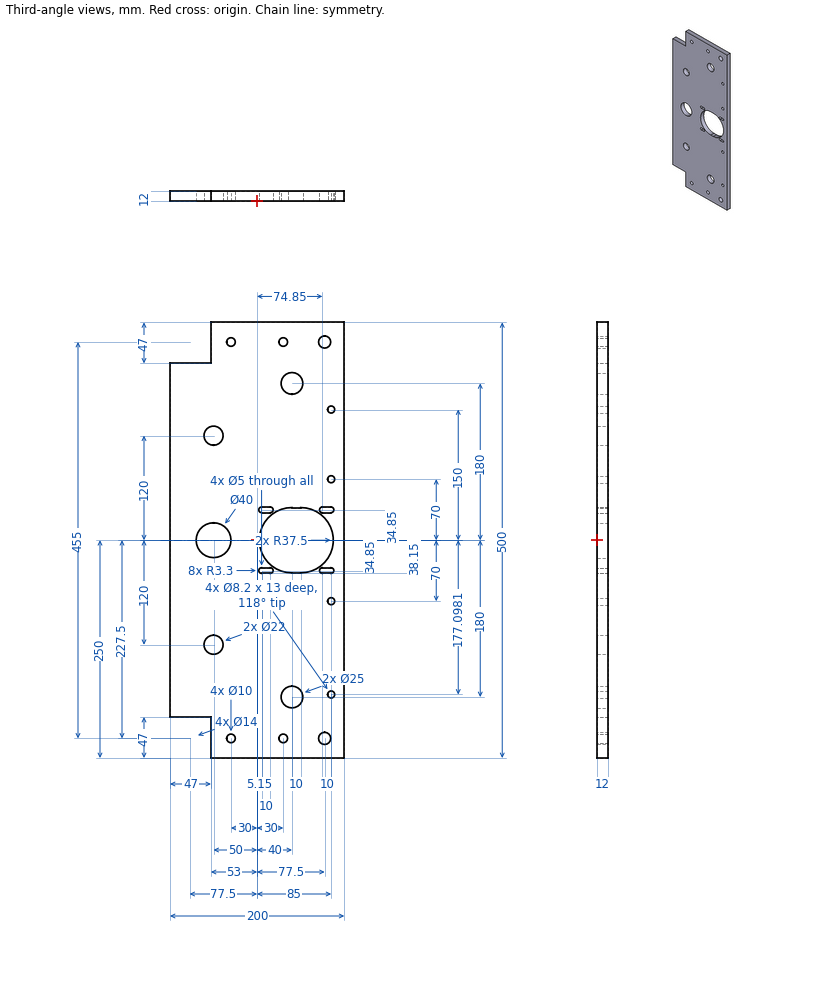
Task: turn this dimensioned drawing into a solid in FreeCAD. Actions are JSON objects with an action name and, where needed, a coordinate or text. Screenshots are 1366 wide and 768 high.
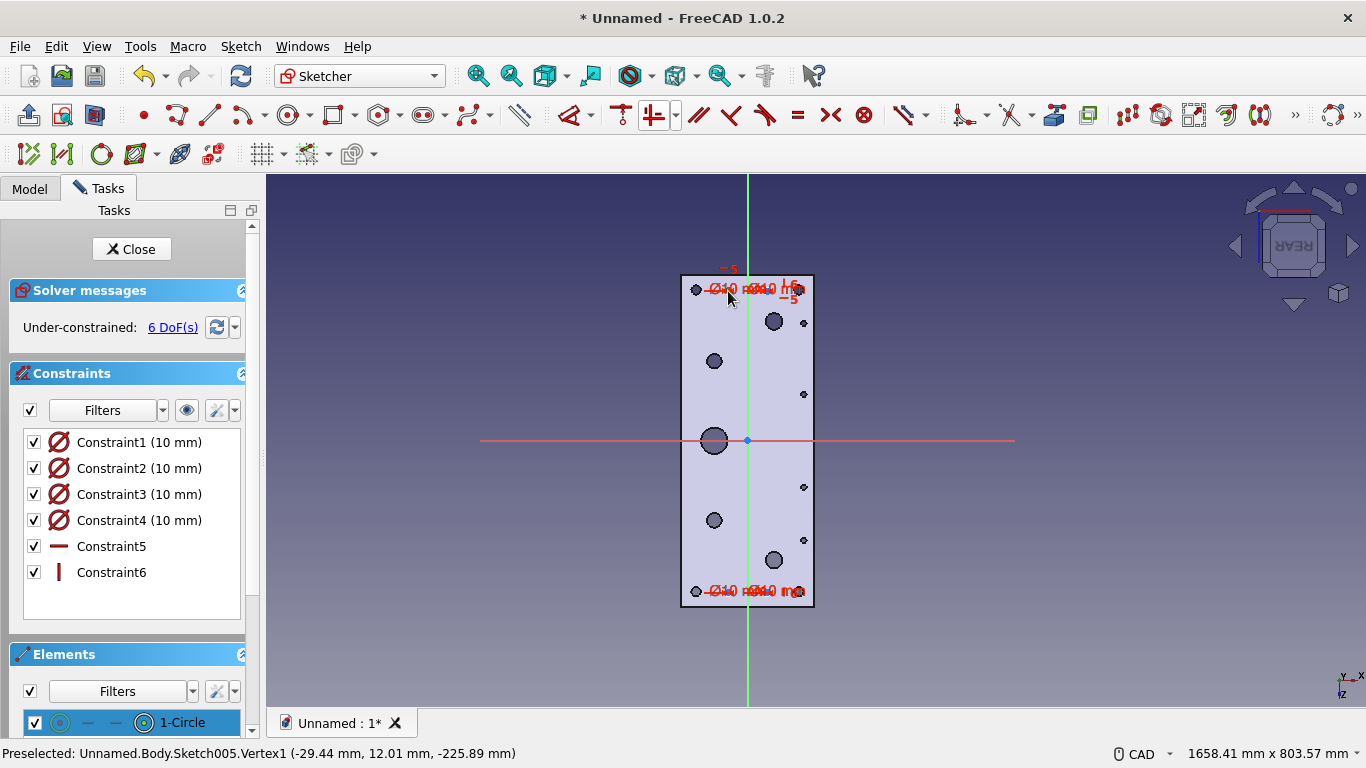
{"action": "left_click", "coordinate": [728, 593]}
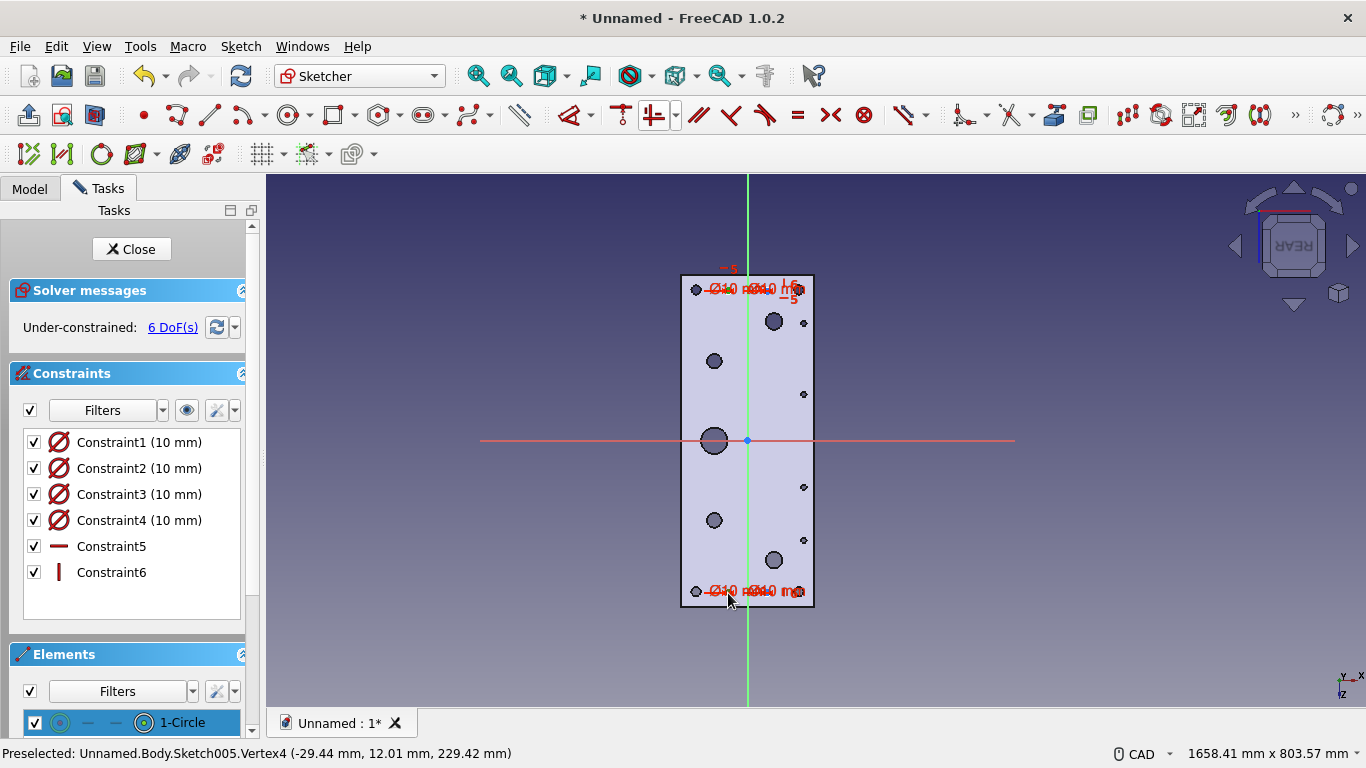
{"action": "key", "text": "v"}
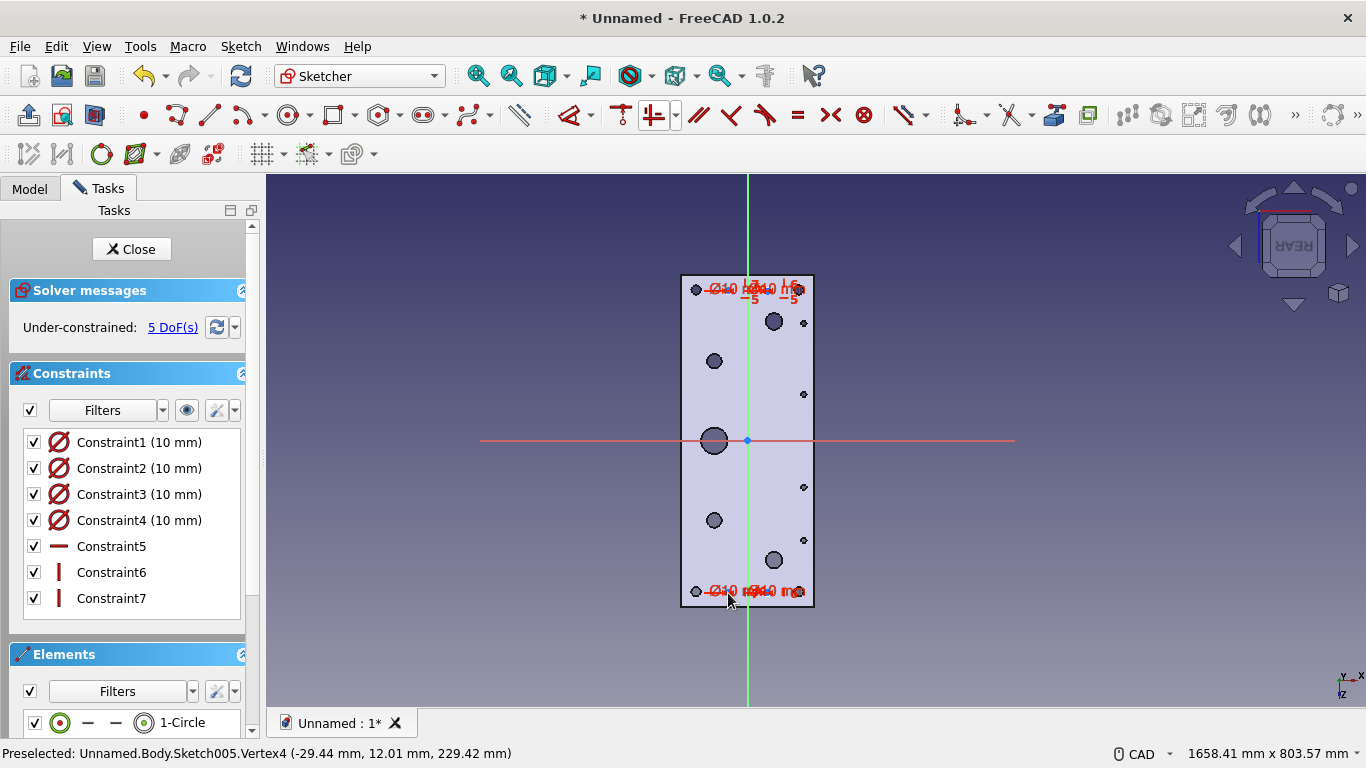
{"action": "left_click", "coordinate": [767, 593]}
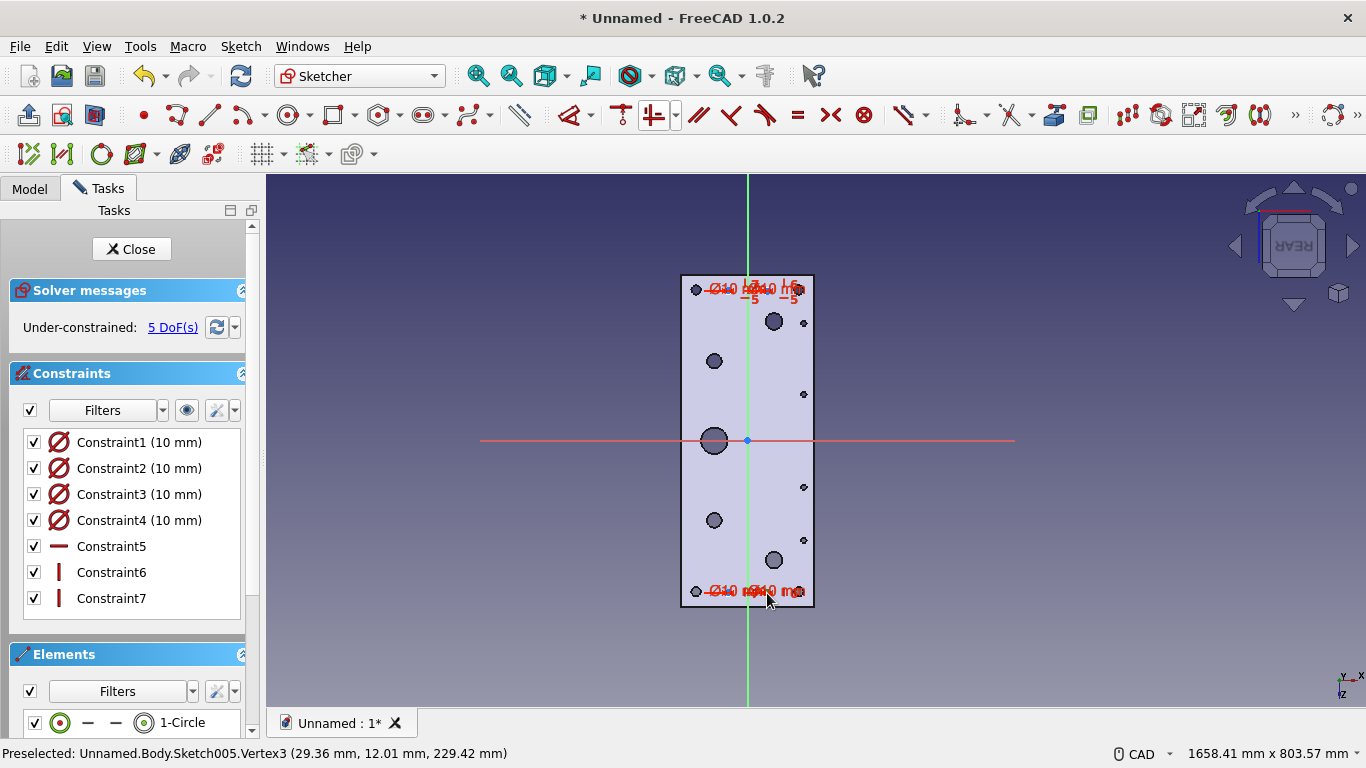
{"action": "left_click", "coordinate": [728, 593]}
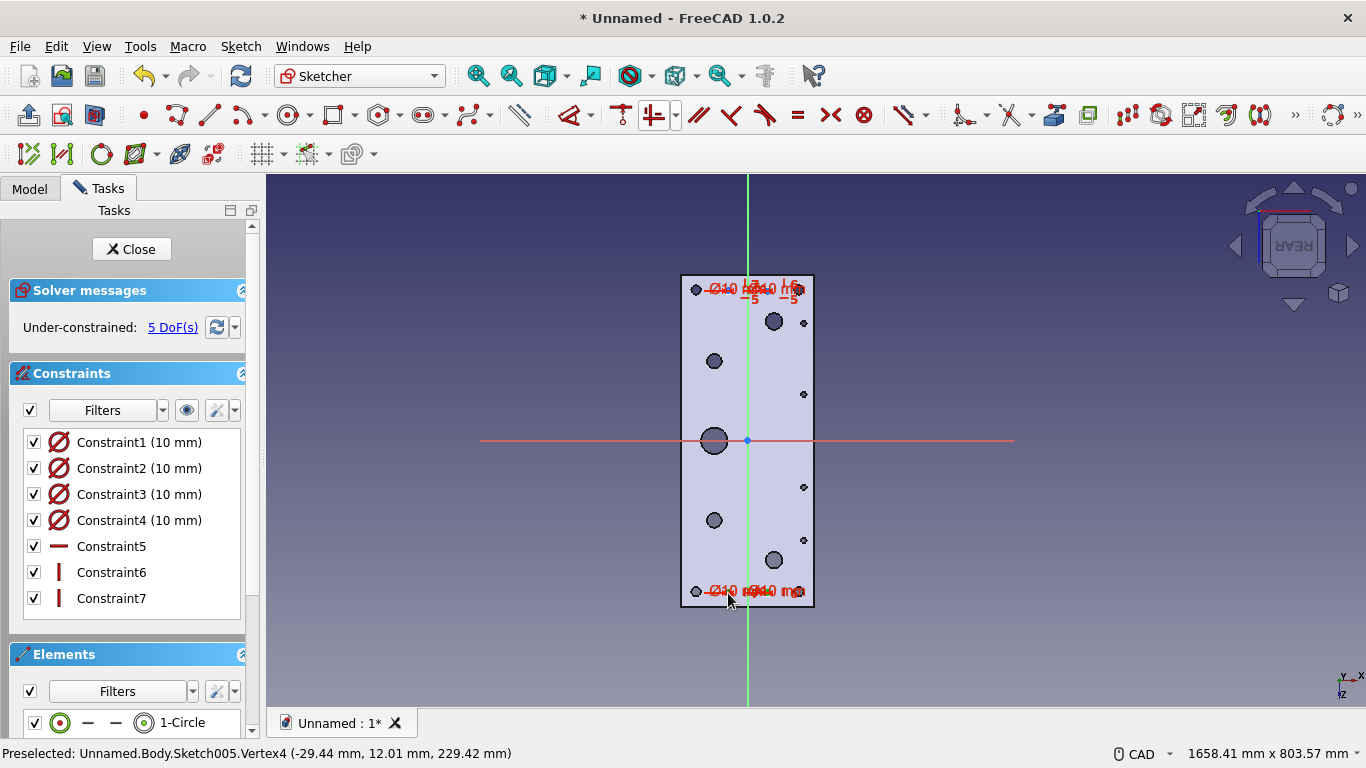
{"action": "key", "text": "h"}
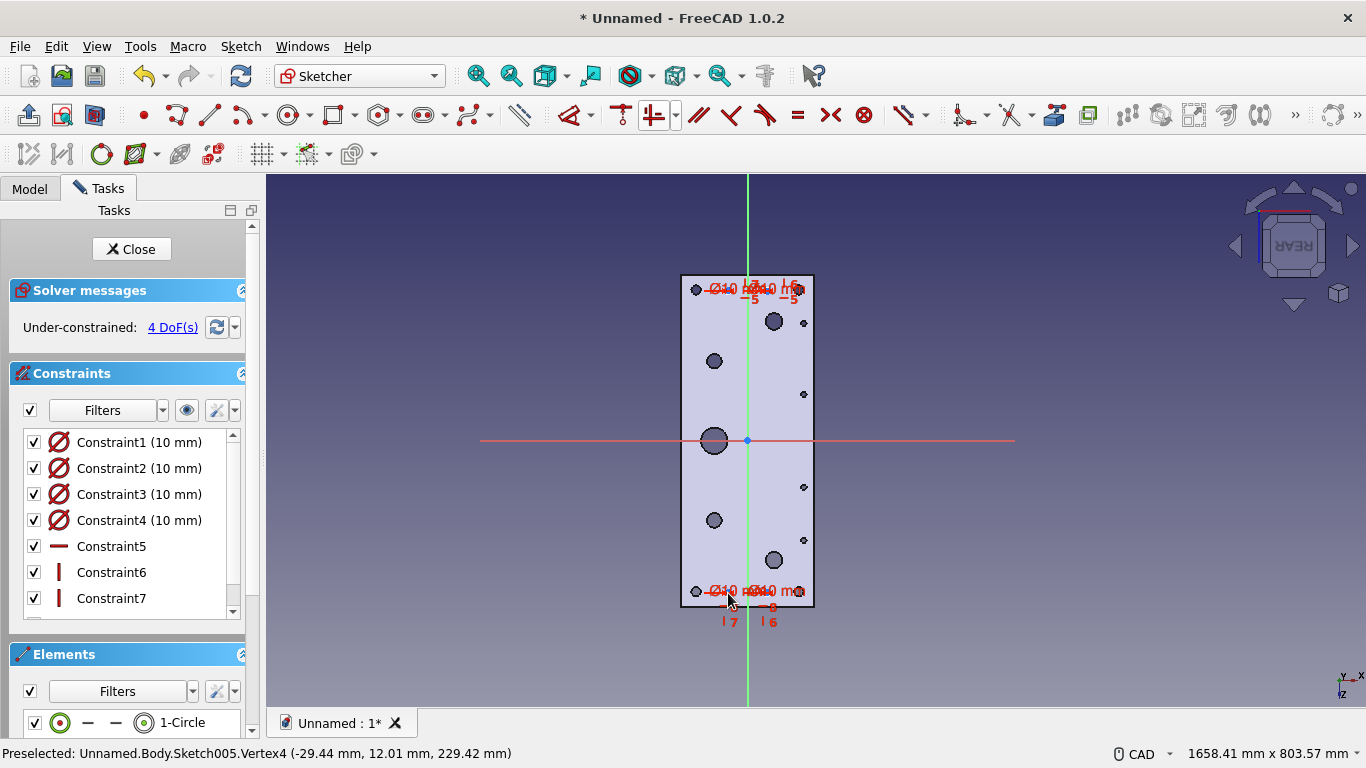
{"action": "key", "text": "d"}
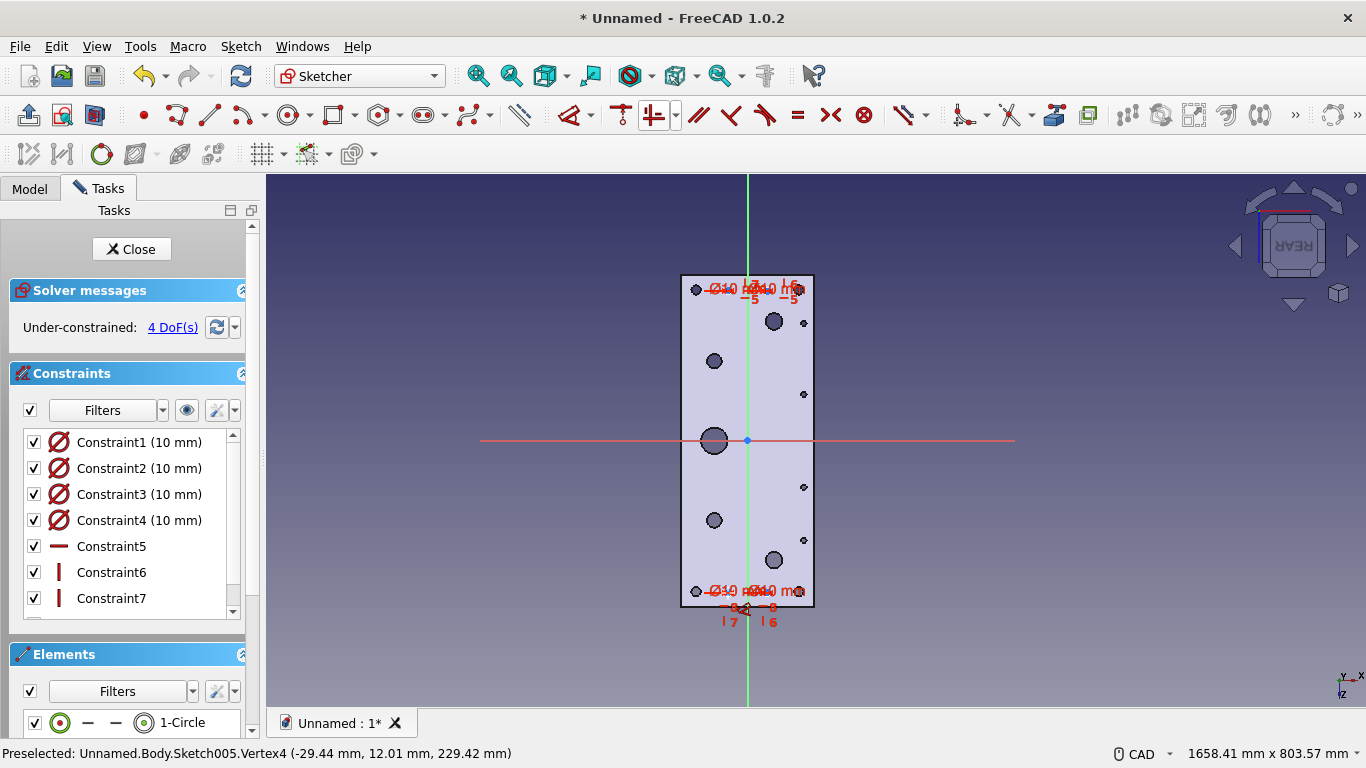
{"action": "scroll", "coordinate": [728, 291], "scroll_direction": "up", "scroll_amount": 4}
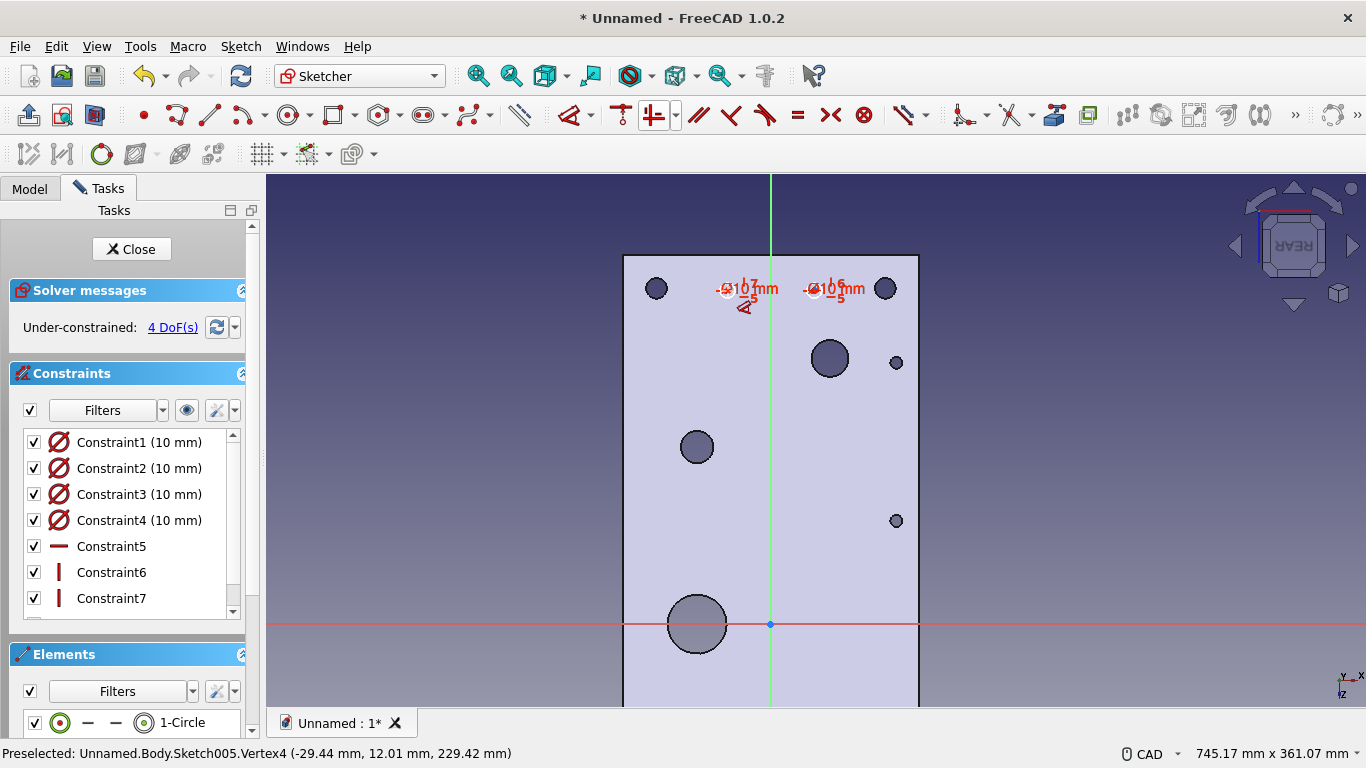
{"action": "left_click", "coordinate": [727, 291]}
{"action": "left_click", "coordinate": [749, 257]}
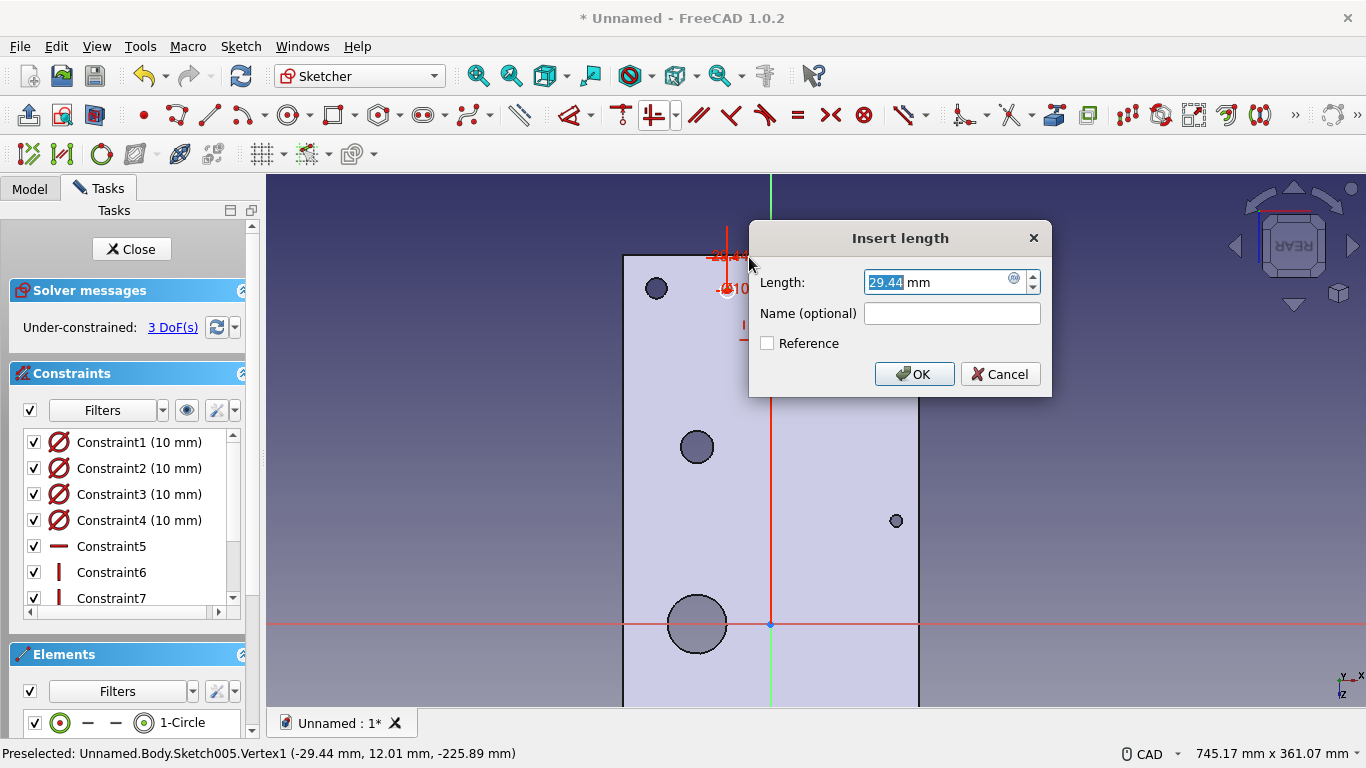
{"action": "type", "text": "30"}
{"action": "key", "text": "Return"}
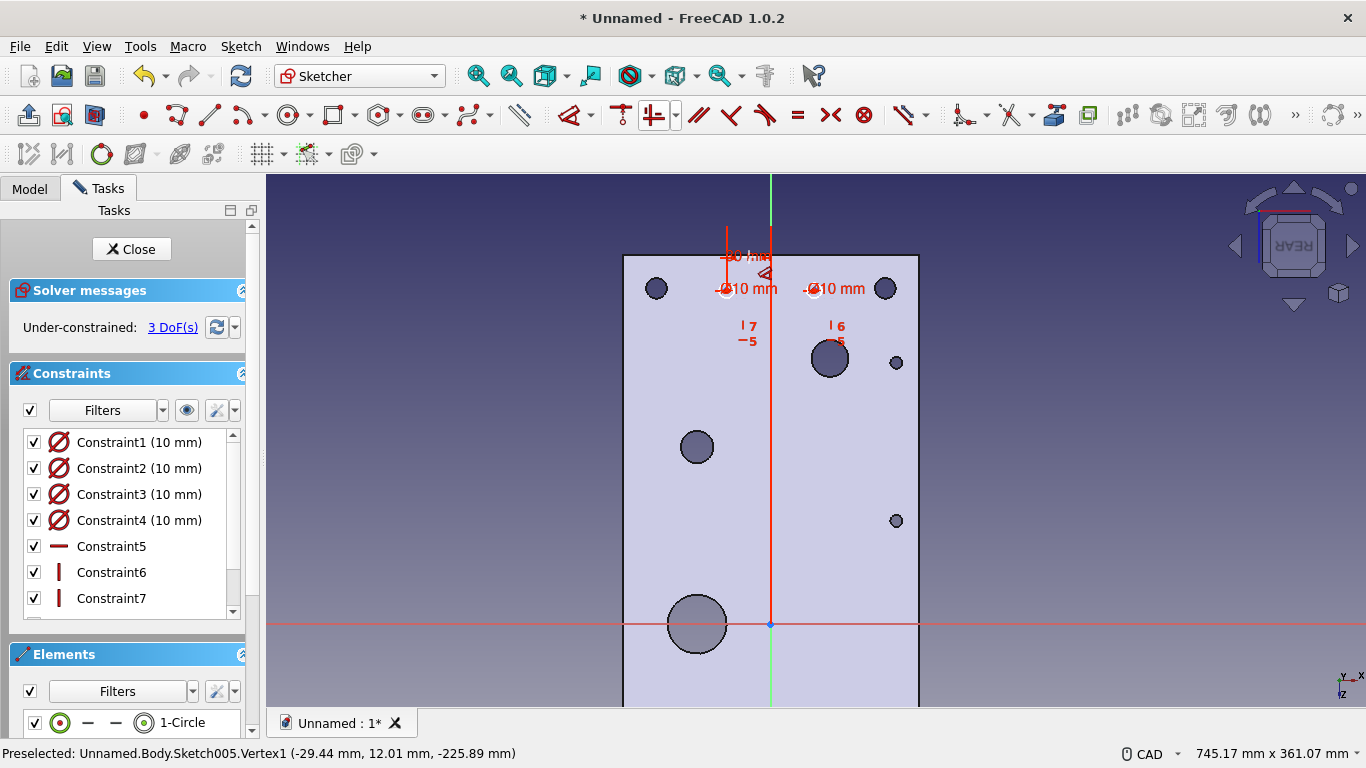
{"action": "left_click", "coordinate": [814, 291]}
{"action": "left_click", "coordinate": [793, 658]}